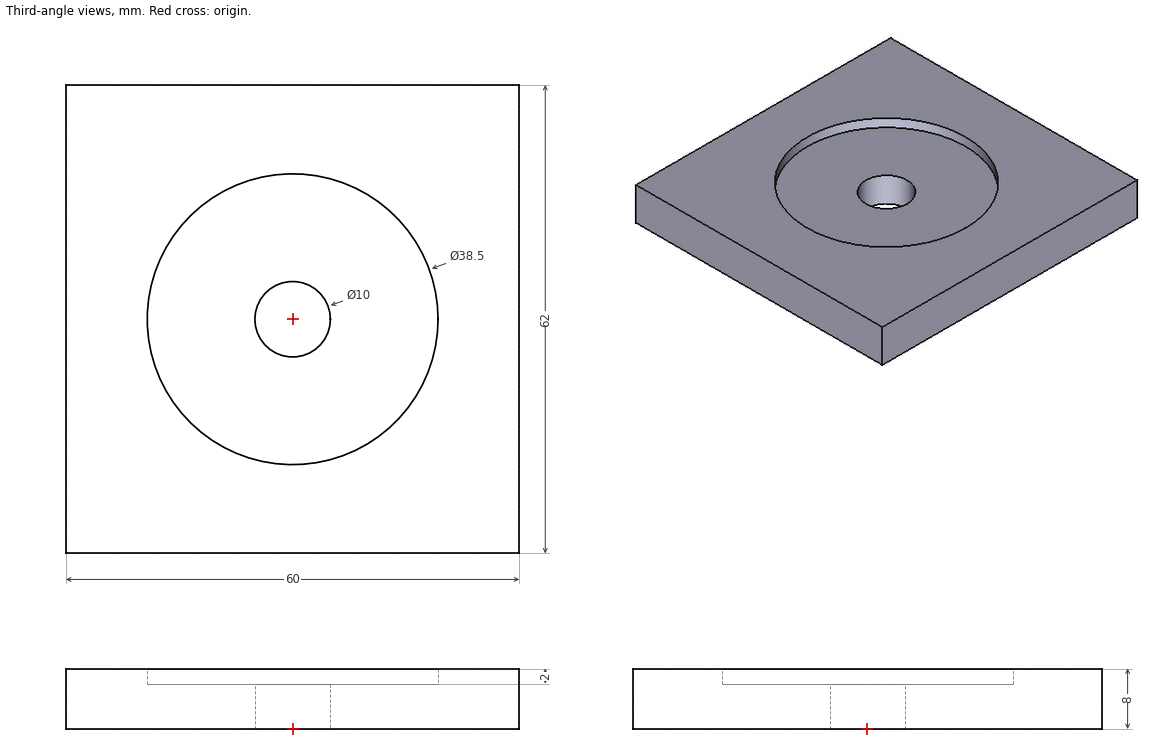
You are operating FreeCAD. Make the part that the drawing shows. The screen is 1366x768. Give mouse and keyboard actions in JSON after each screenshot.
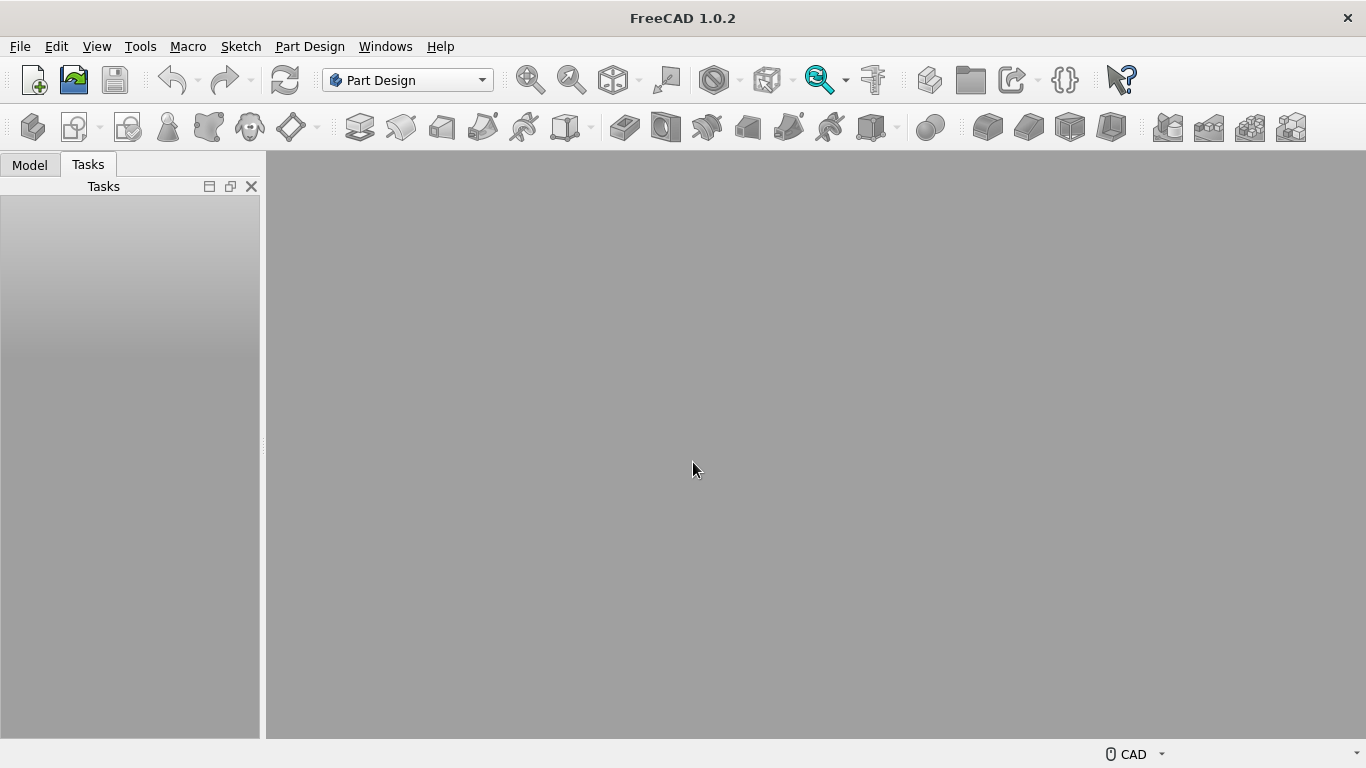
{"action": "left_click", "coordinate": [33, 80]}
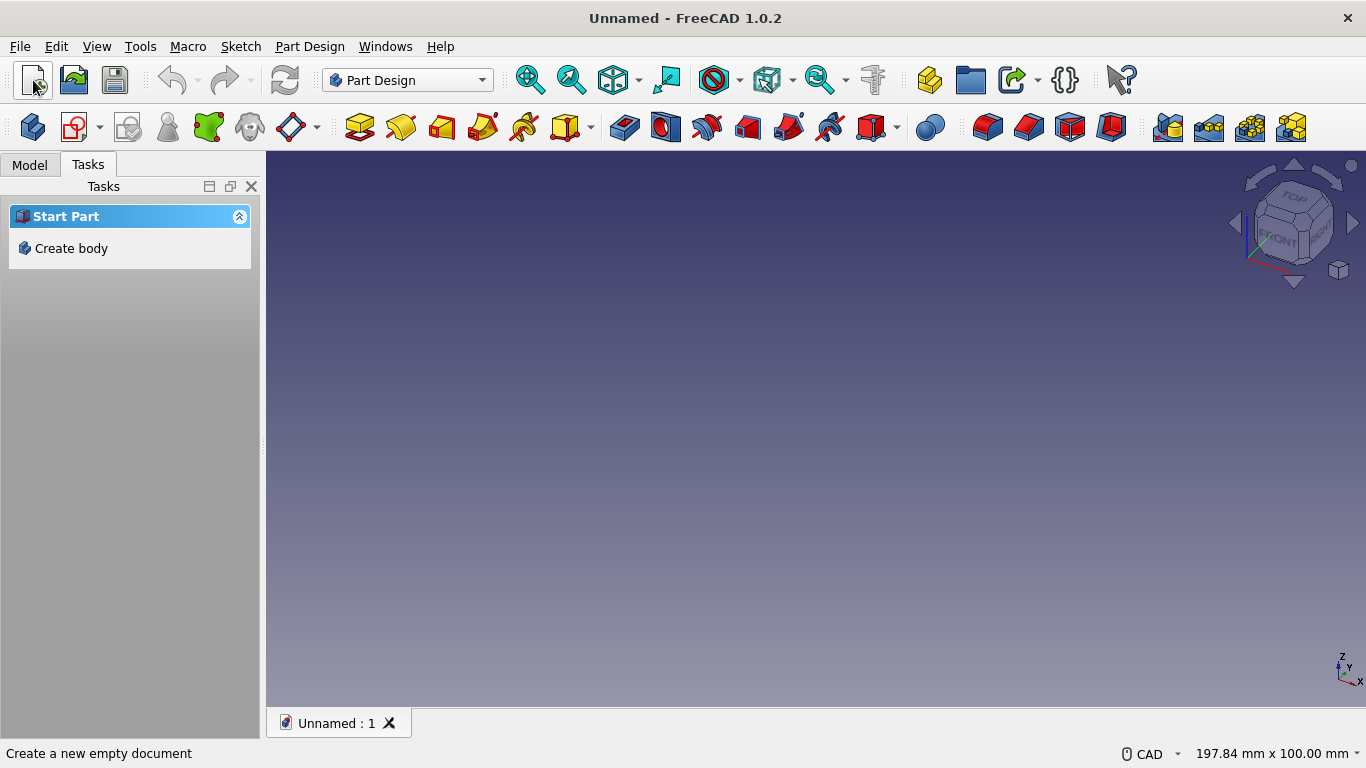
{"action": "left_click", "coordinate": [74, 128]}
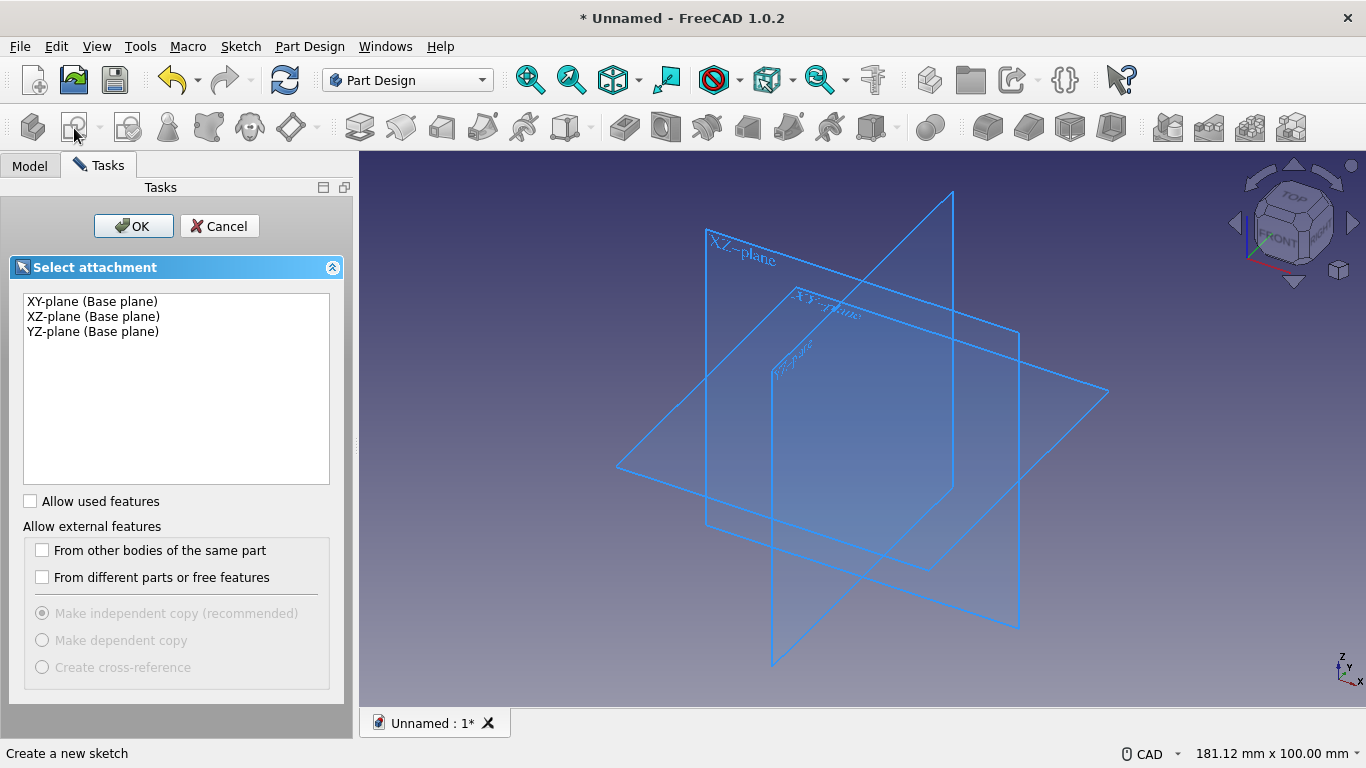
{"action": "left_click", "coordinate": [84, 302]}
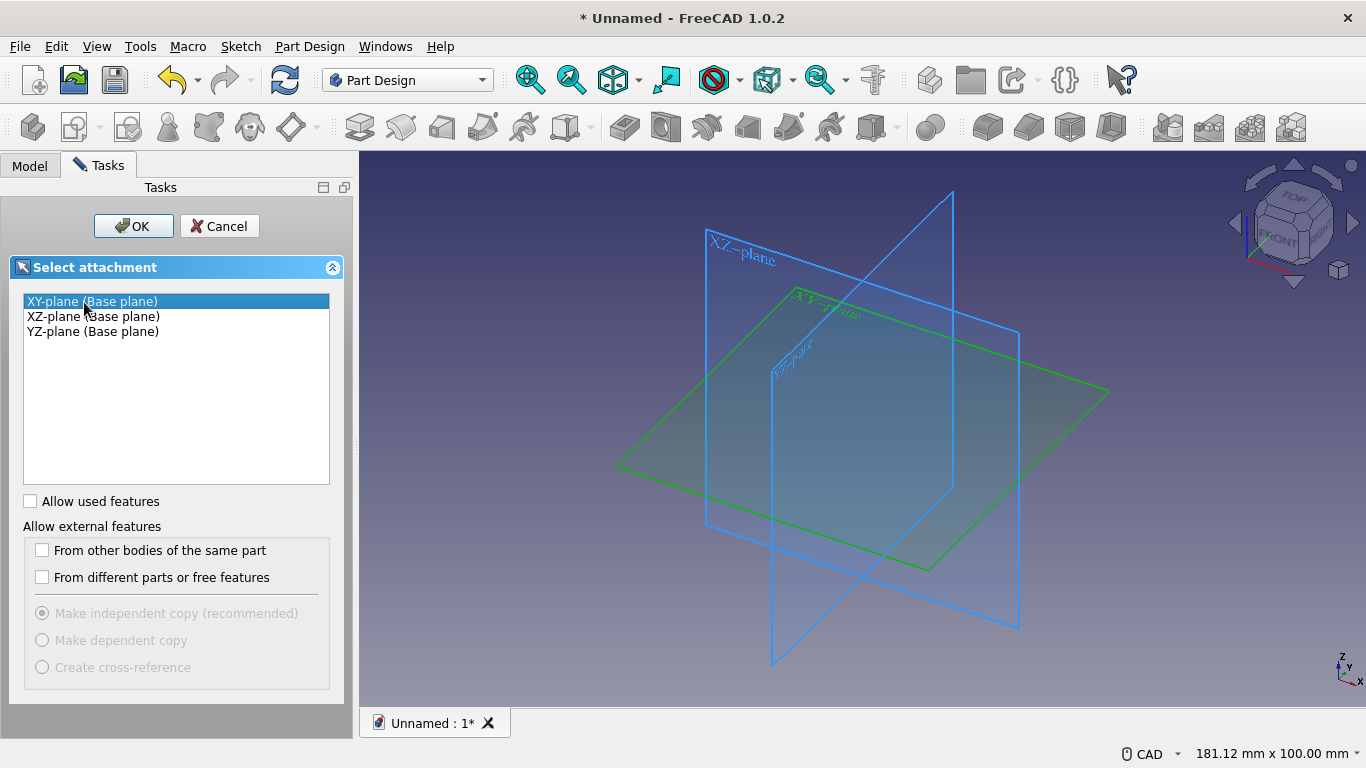
{"action": "left_click", "coordinate": [134, 226]}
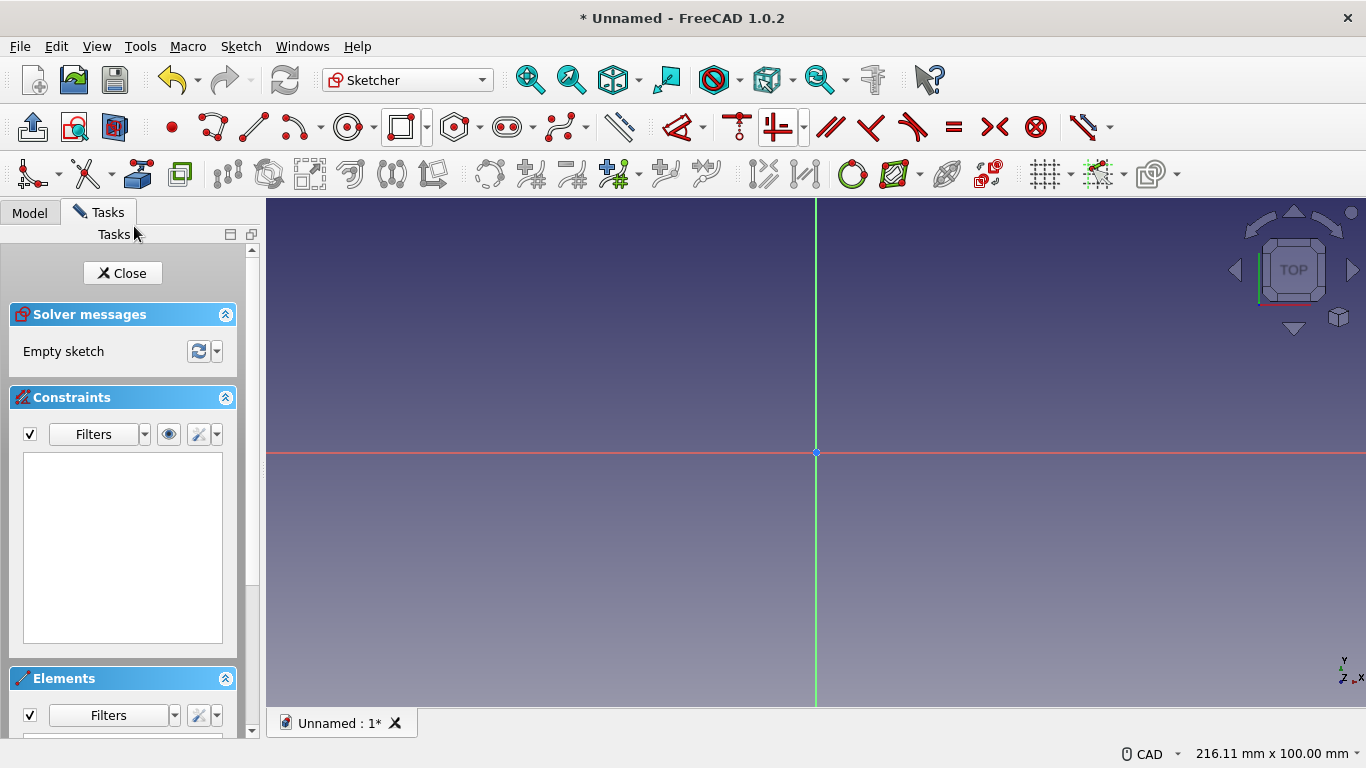
{"action": "key", "text": "g v"}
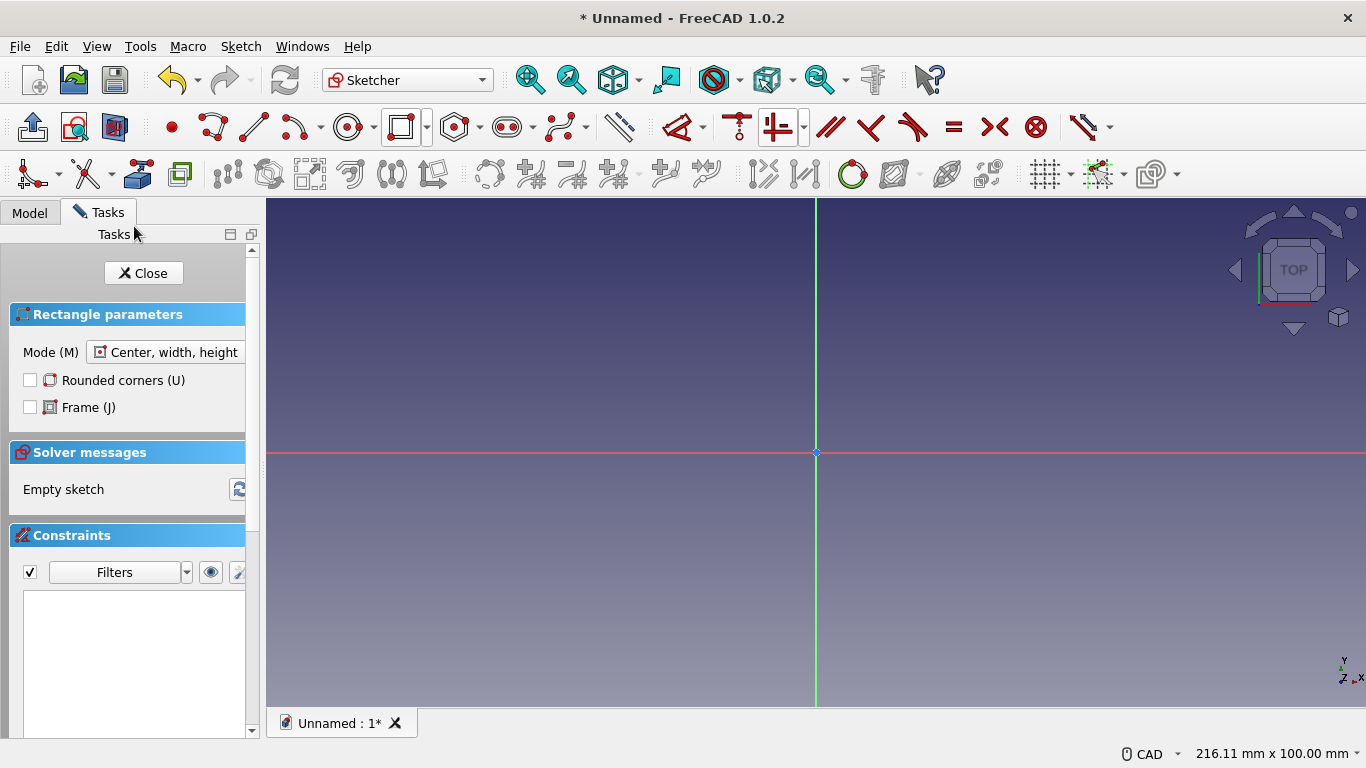
{"action": "left_click", "coordinate": [816, 452]}
{"action": "mouse_move", "coordinate": [969, 295]}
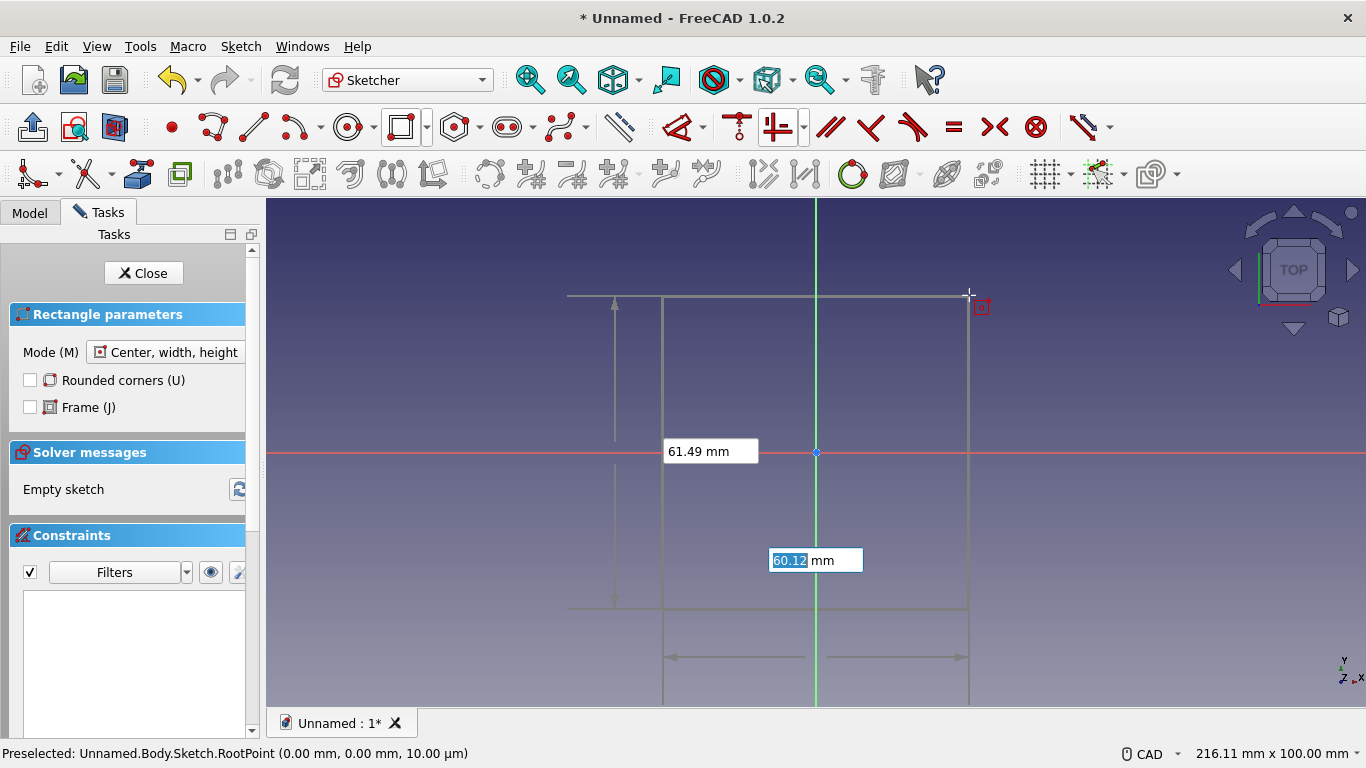
{"action": "type", "text": "60"}
{"action": "key", "text": "Tab"}
{"action": "type", "text": "62"}
{"action": "key", "text": "Return"}
{"action": "key", "text": "Escape"}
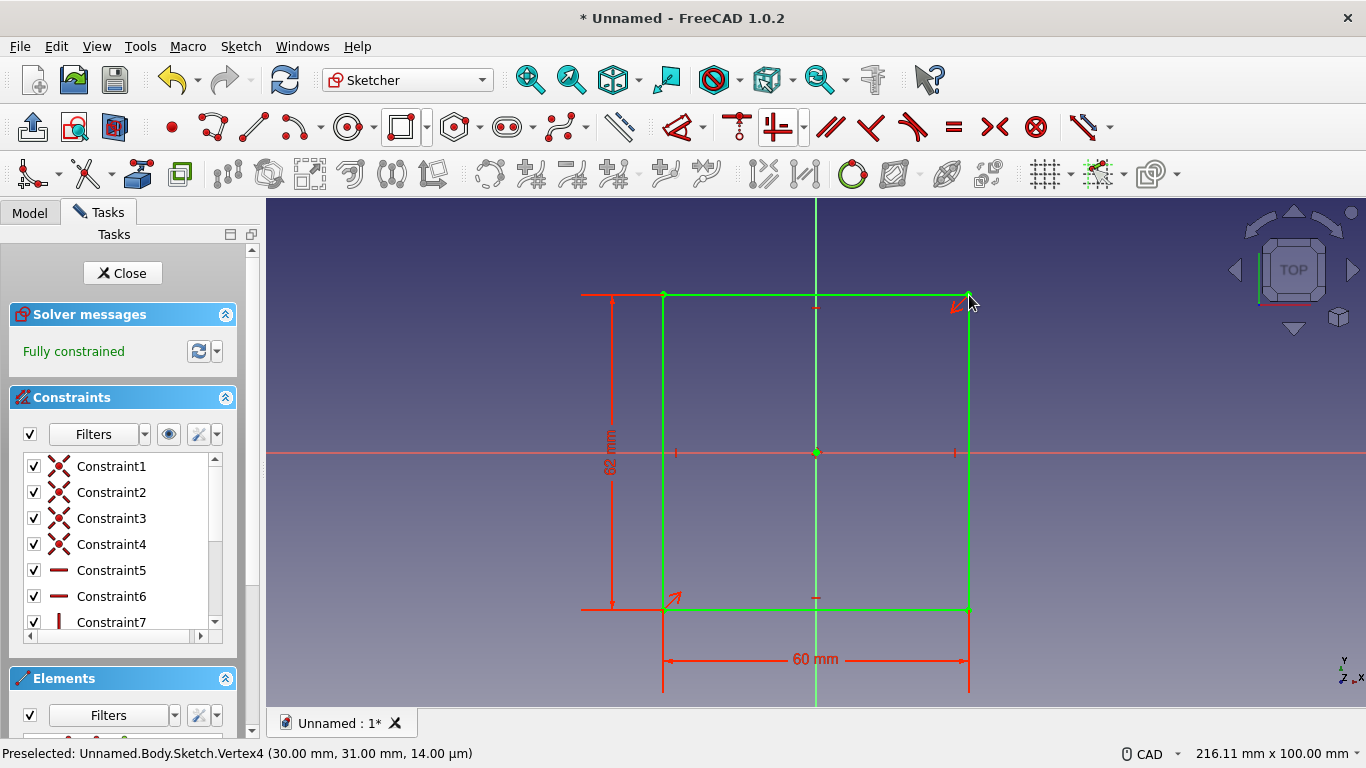
{"action": "left_click", "coordinate": [123, 273]}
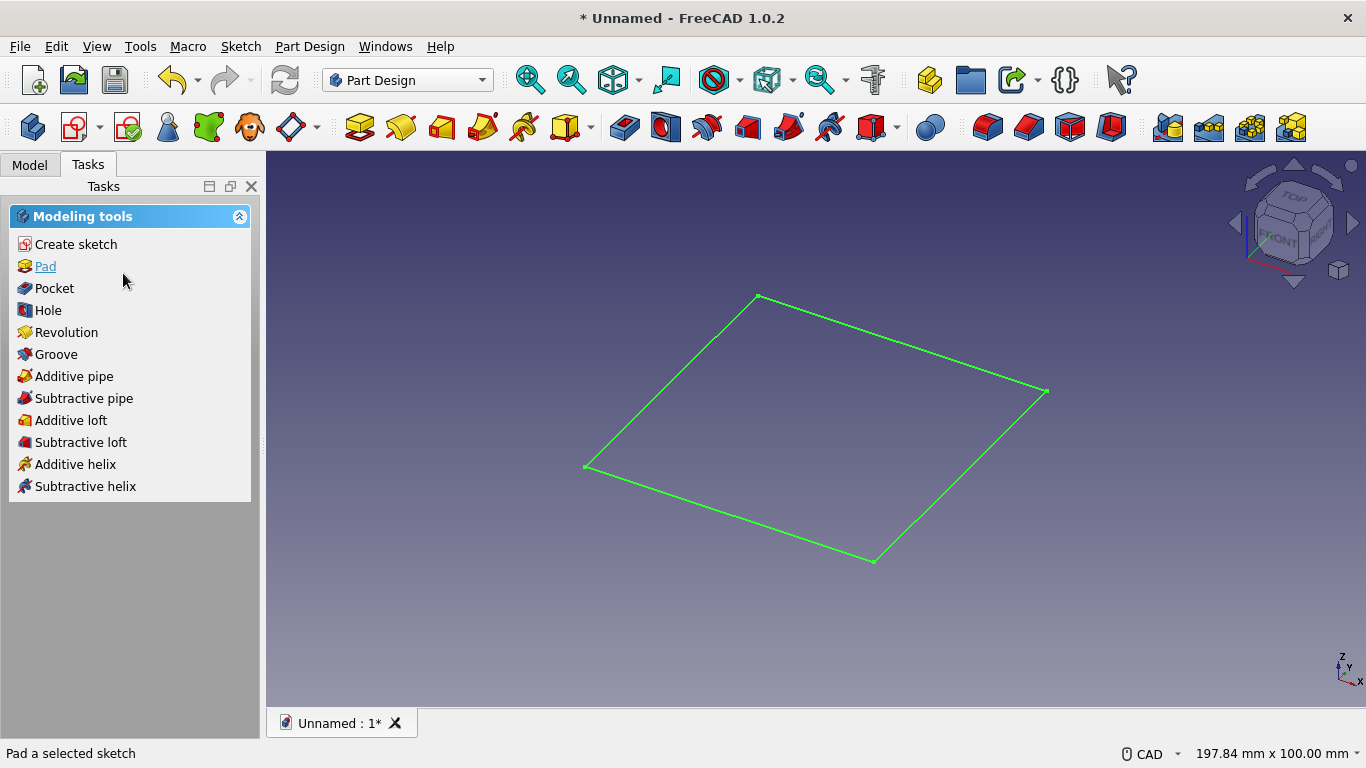
{"action": "left_click", "coordinate": [360, 128]}